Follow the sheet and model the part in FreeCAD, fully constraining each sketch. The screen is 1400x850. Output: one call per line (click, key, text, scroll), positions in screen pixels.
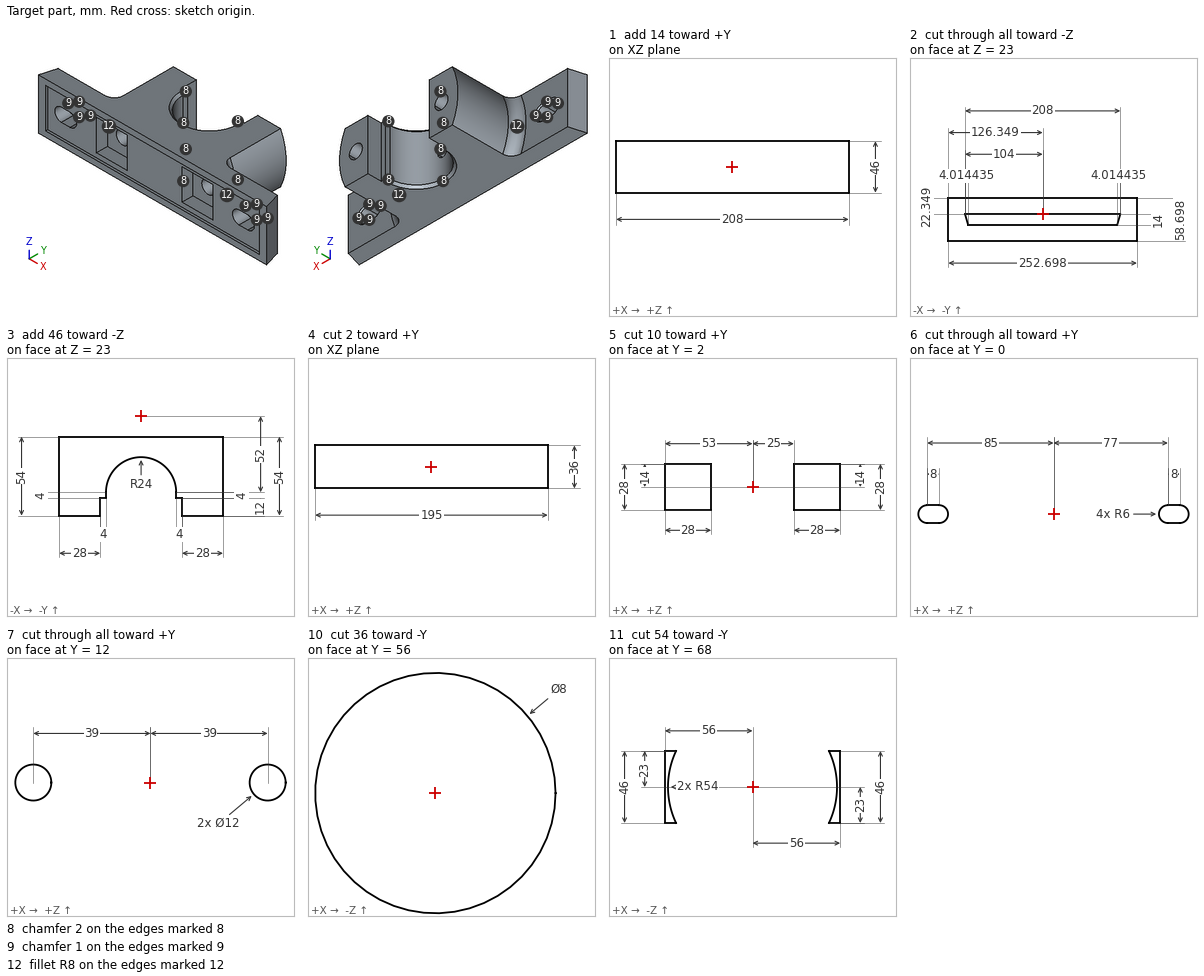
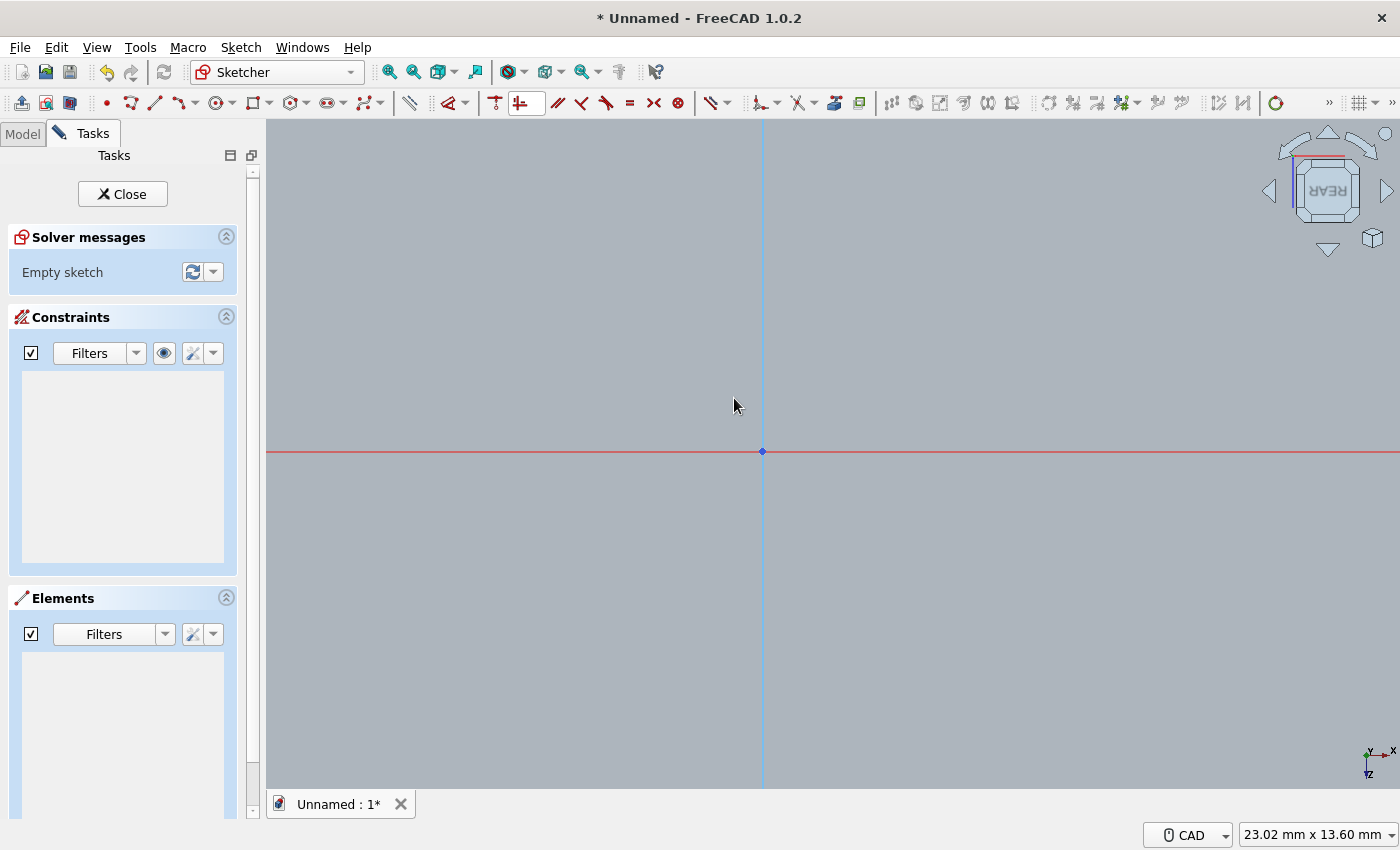
key(g)
key(c)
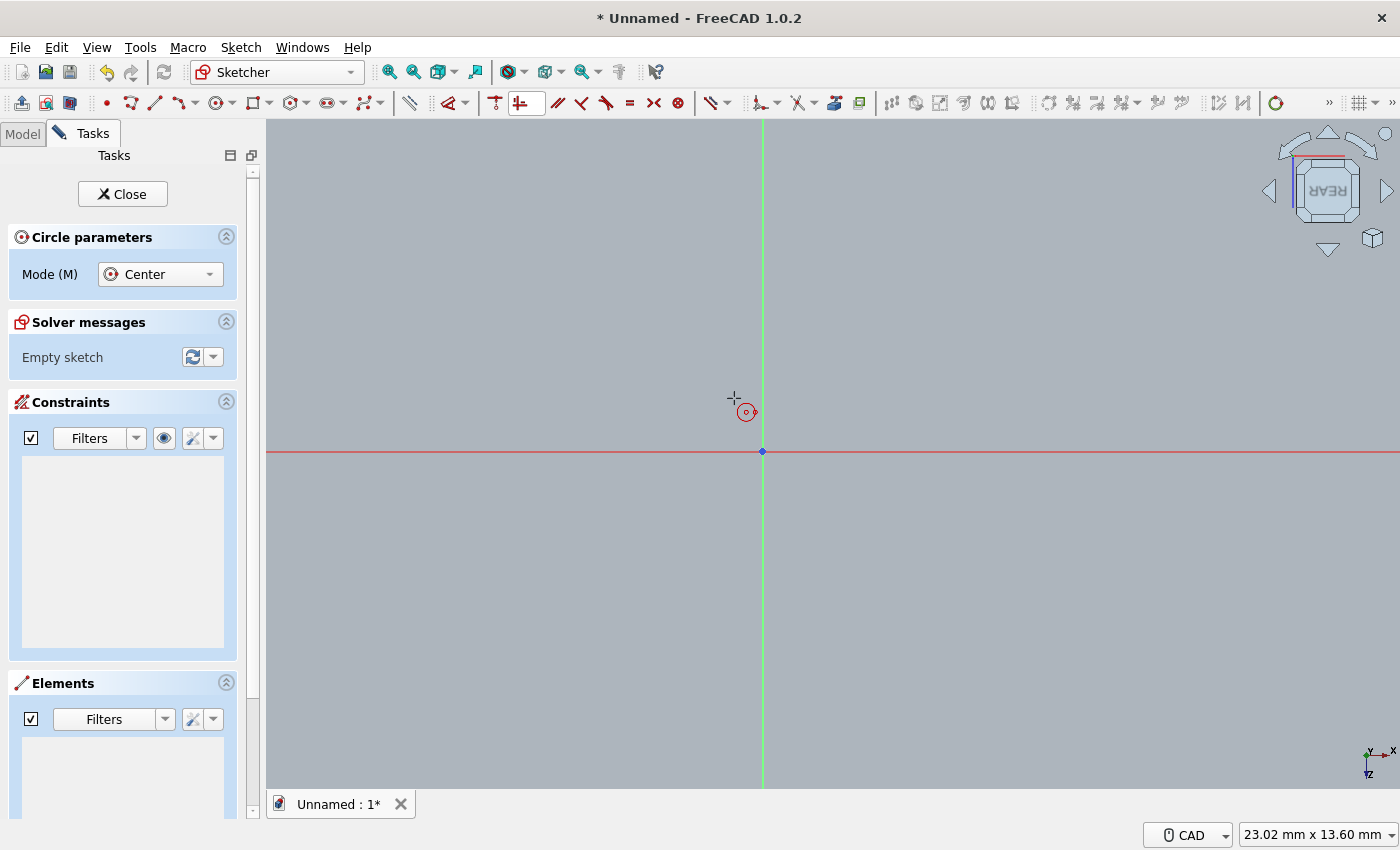
click(763, 452)
move(902, 313)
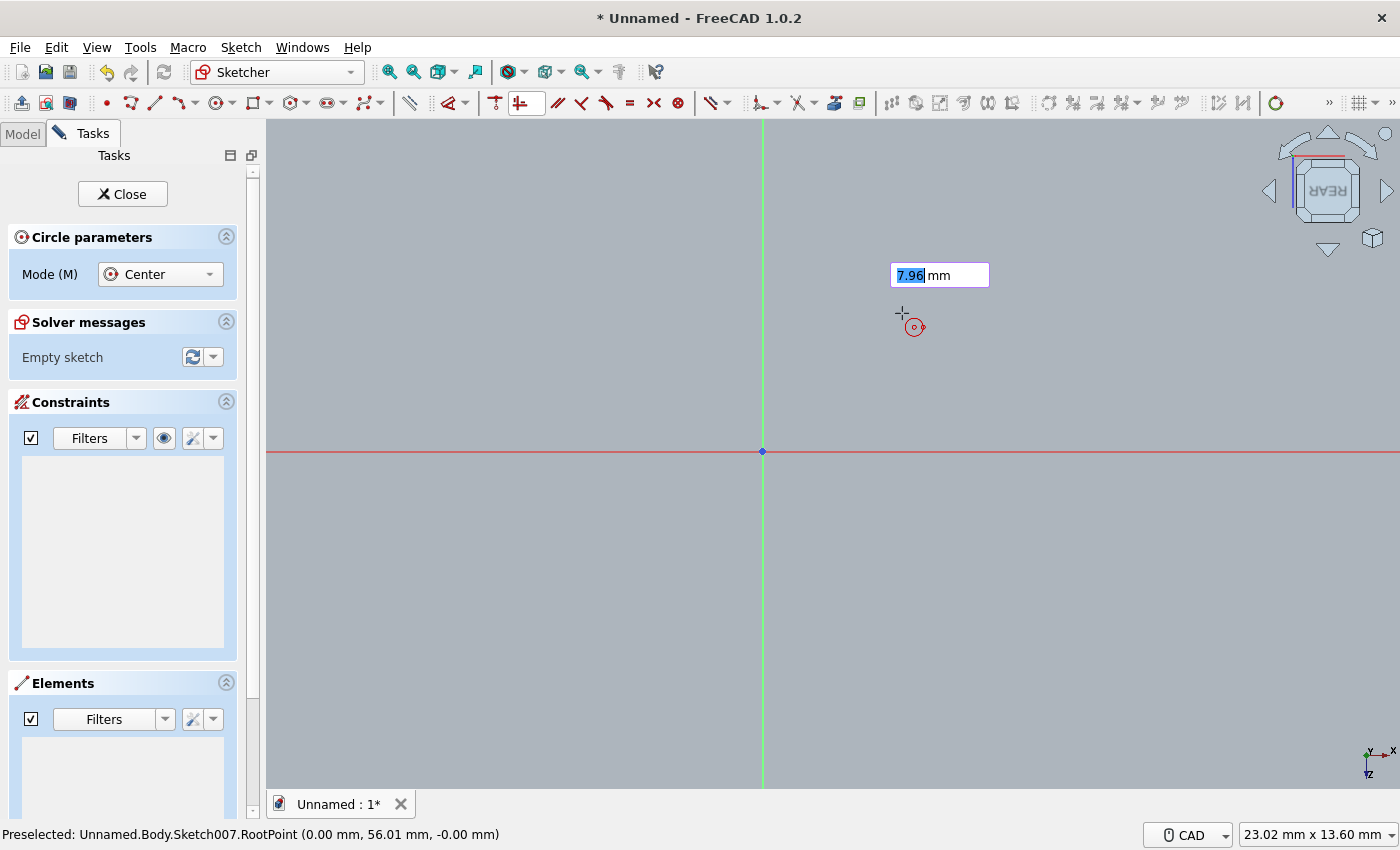
text(8)
key(Return)
key(Escape)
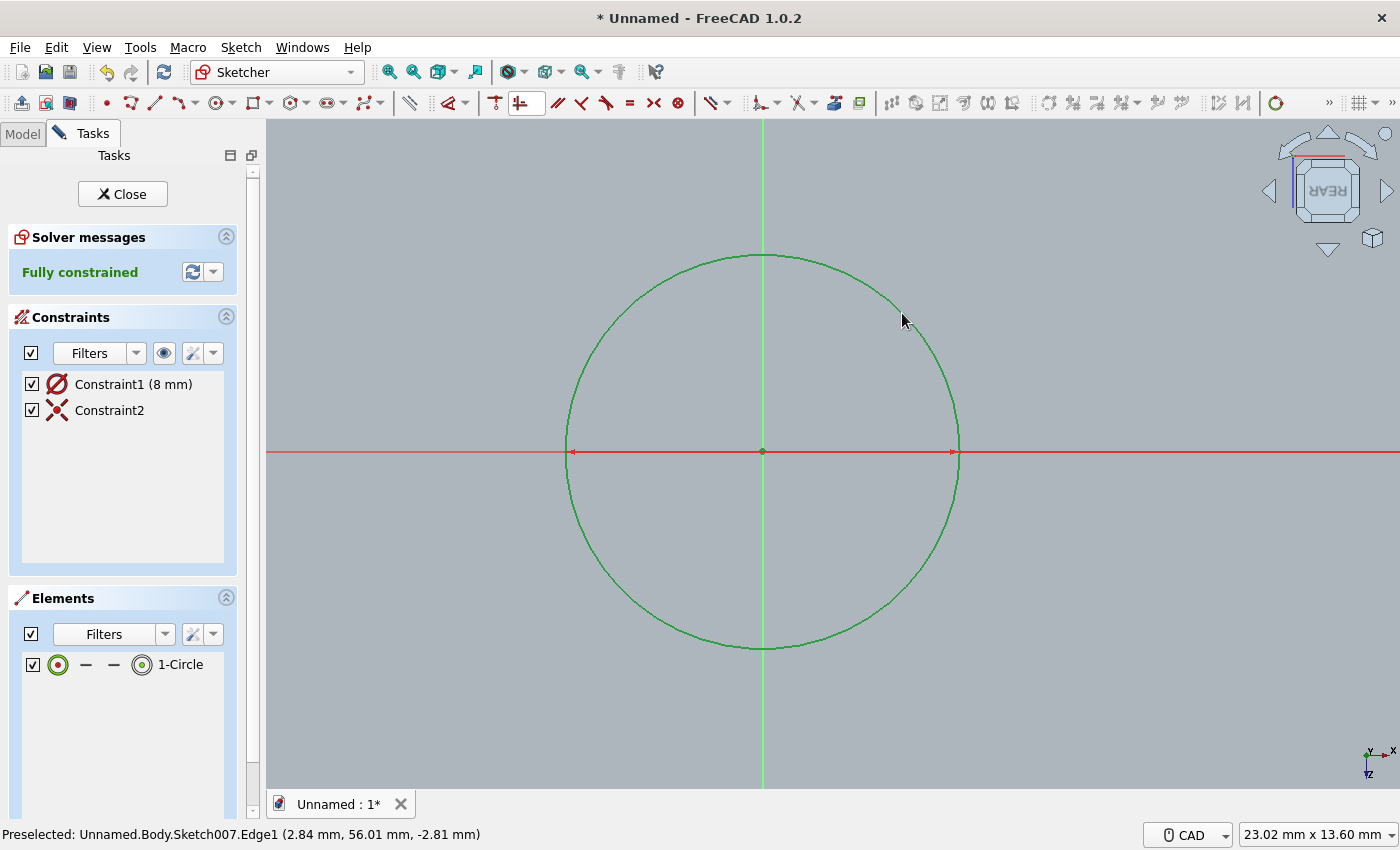
click(123, 194)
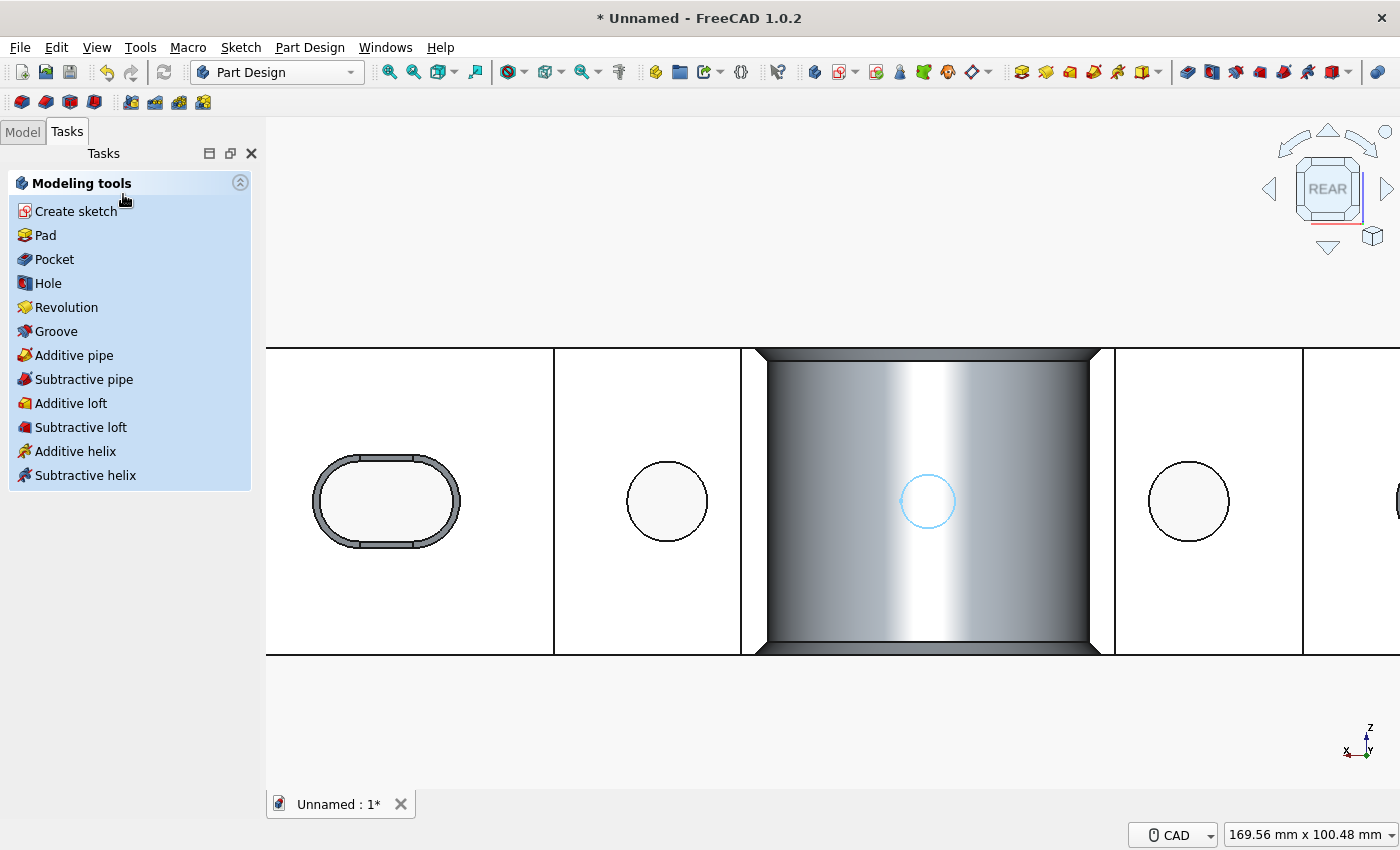
click(1188, 72)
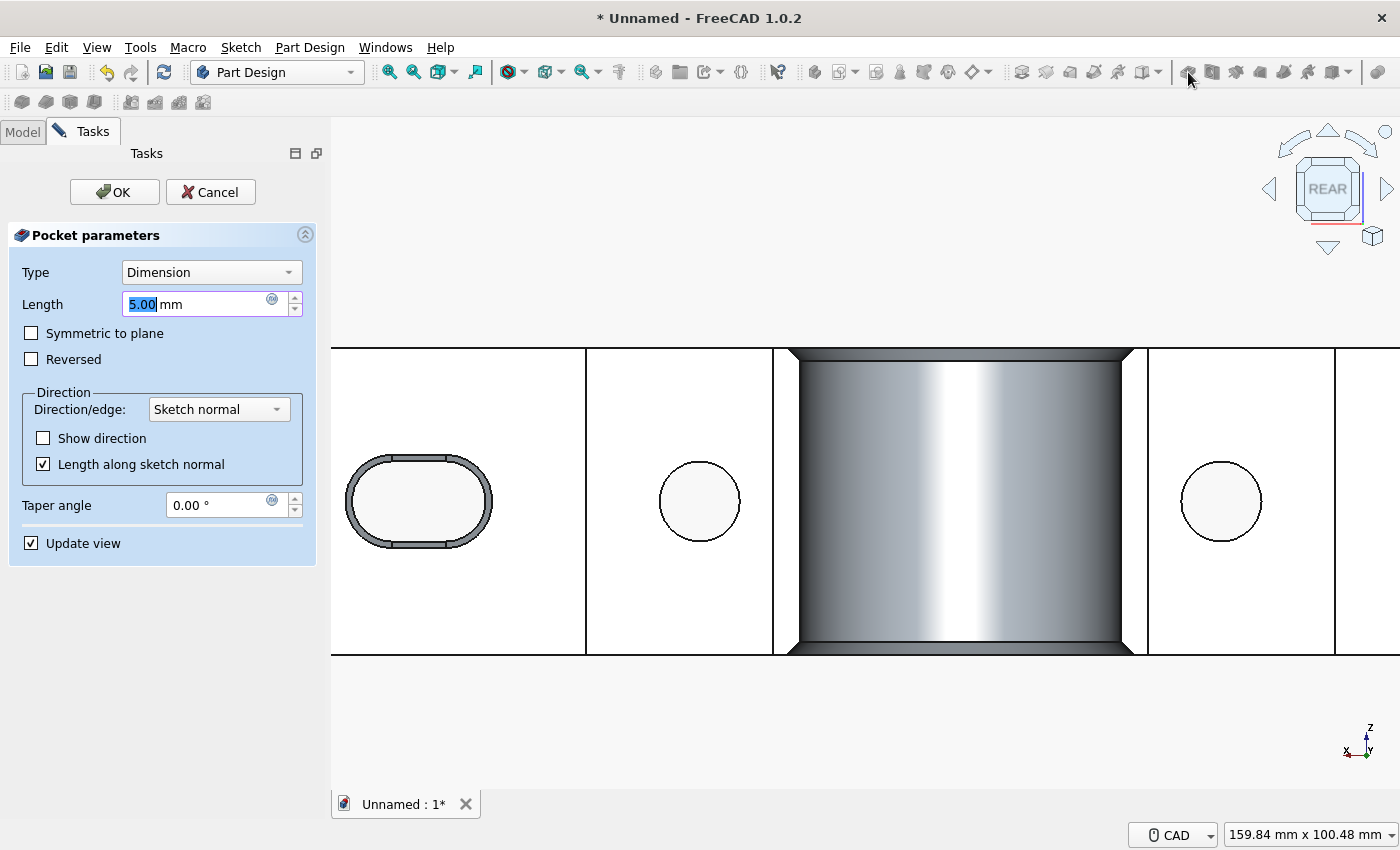
text(36)
key(Tab)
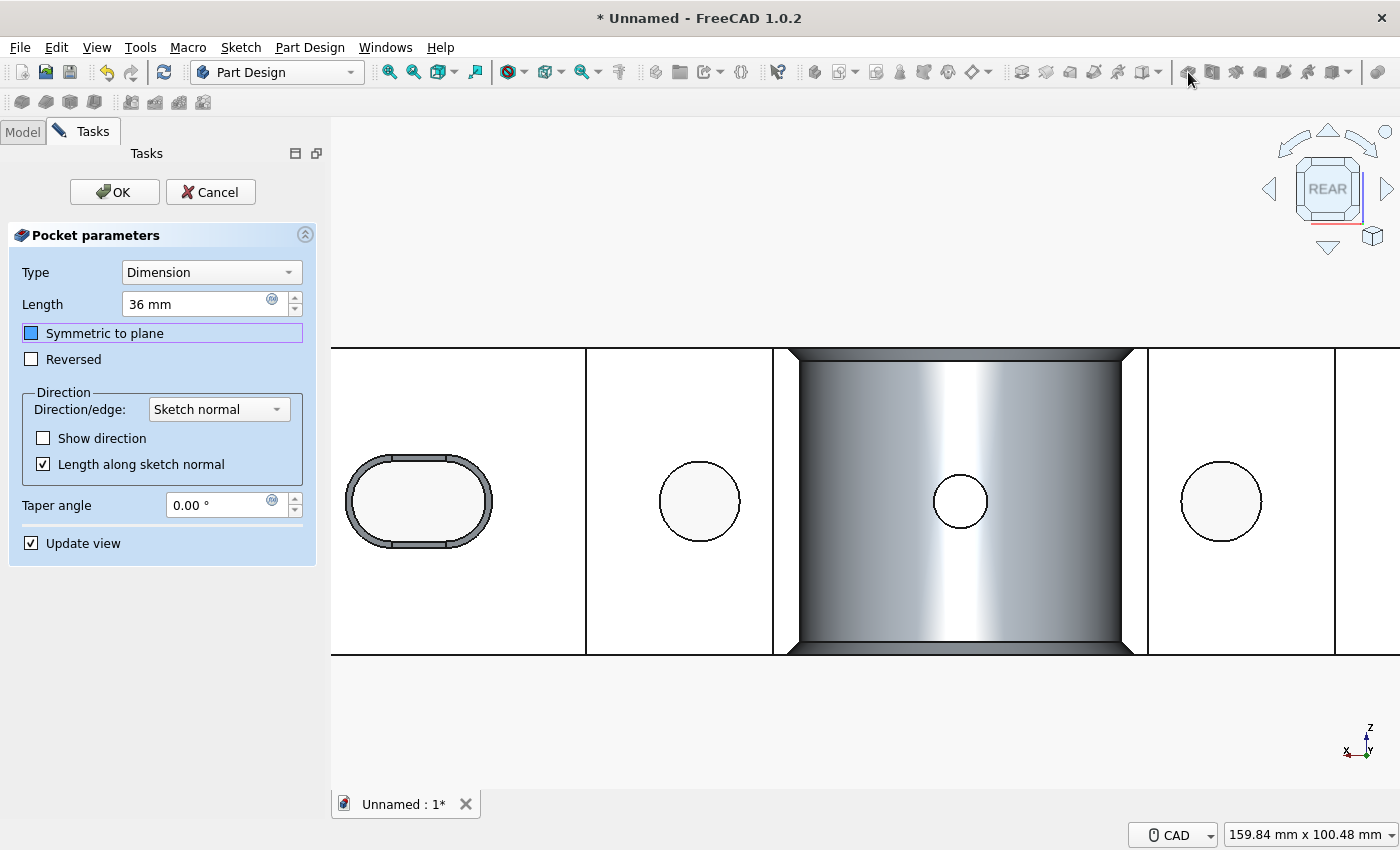
click(115, 192)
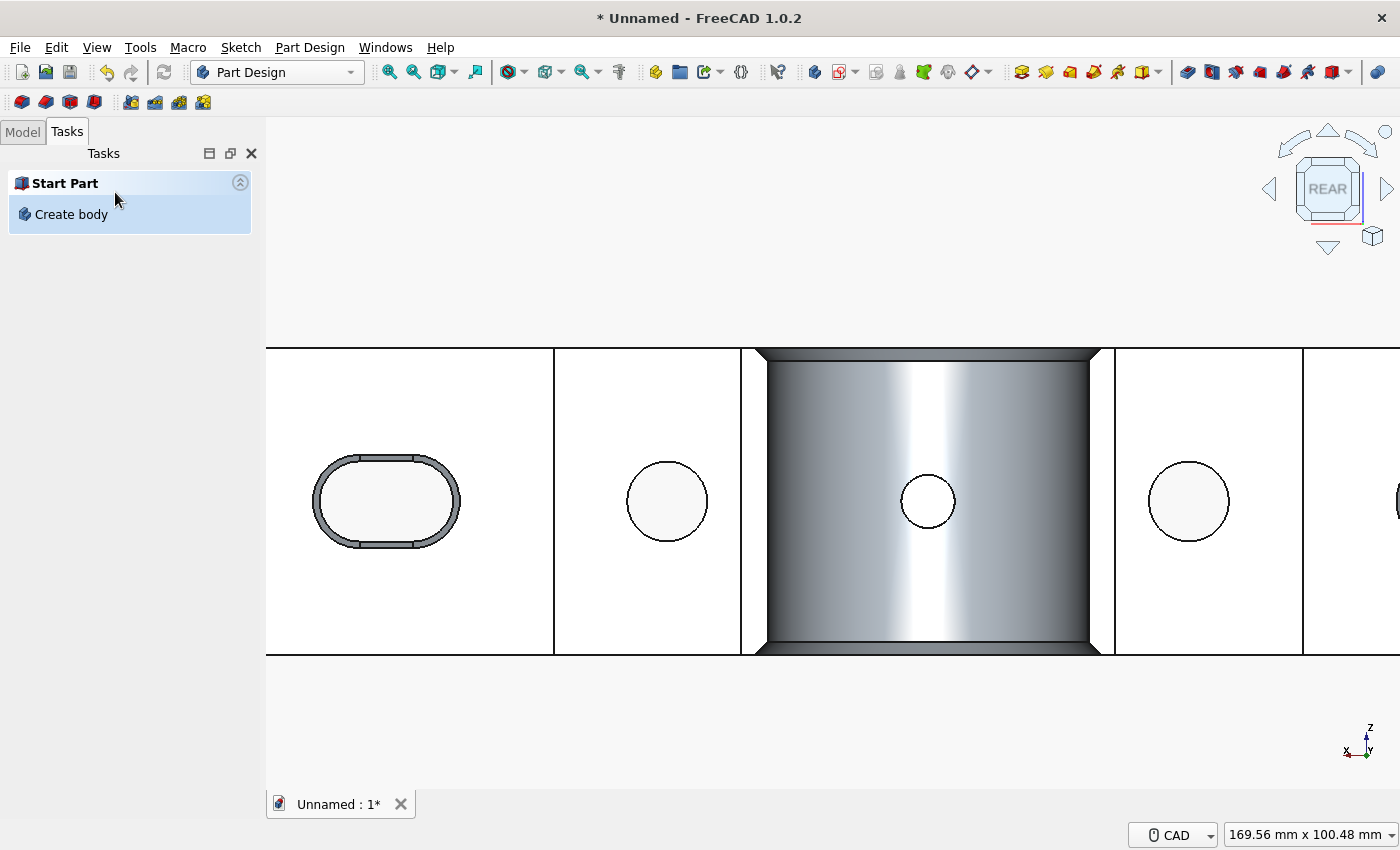
click(390, 72)